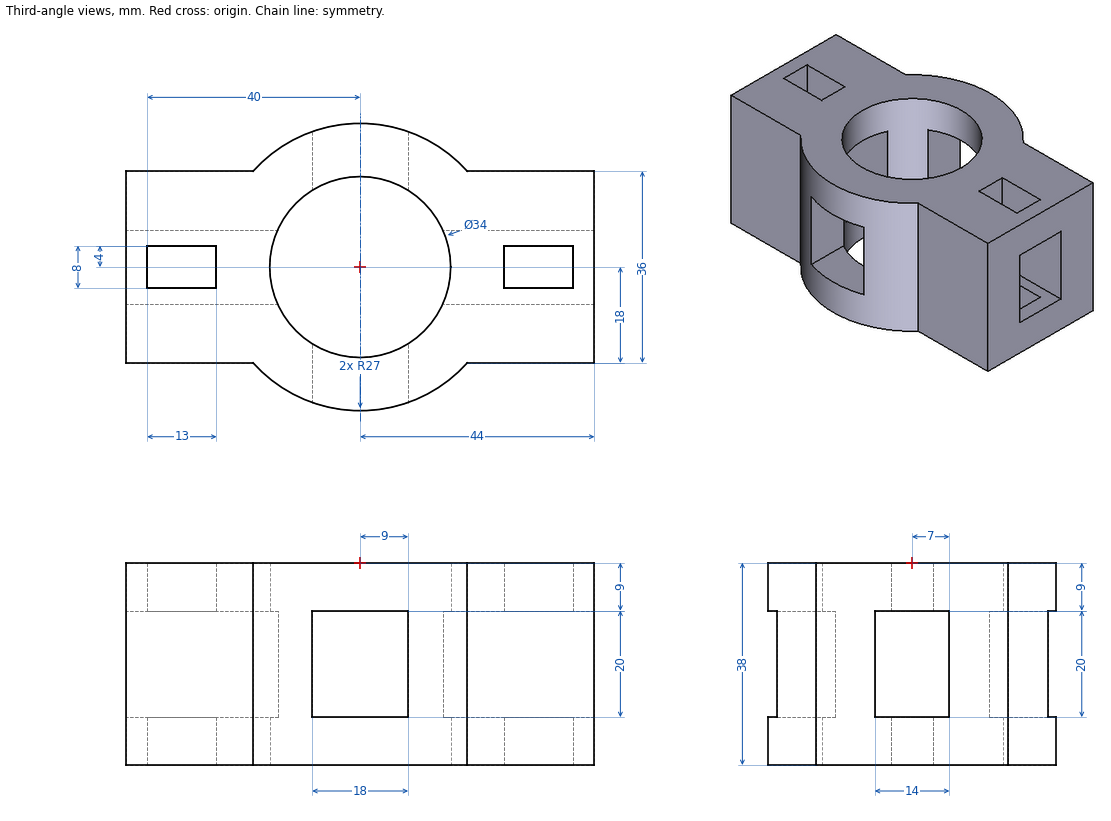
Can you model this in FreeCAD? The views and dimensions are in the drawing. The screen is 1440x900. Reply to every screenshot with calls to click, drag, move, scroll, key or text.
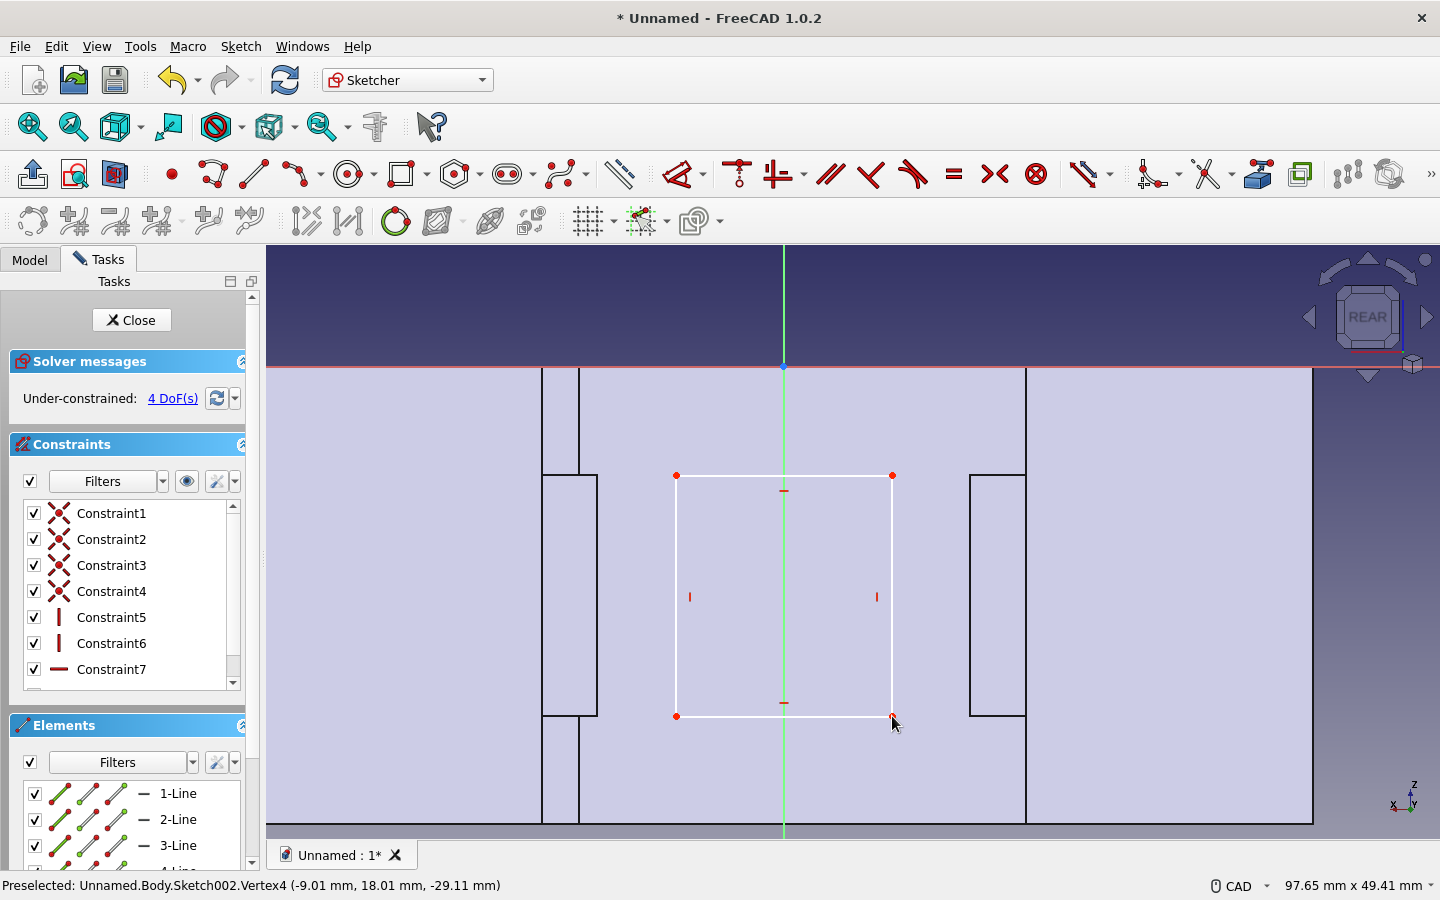
click(676, 174)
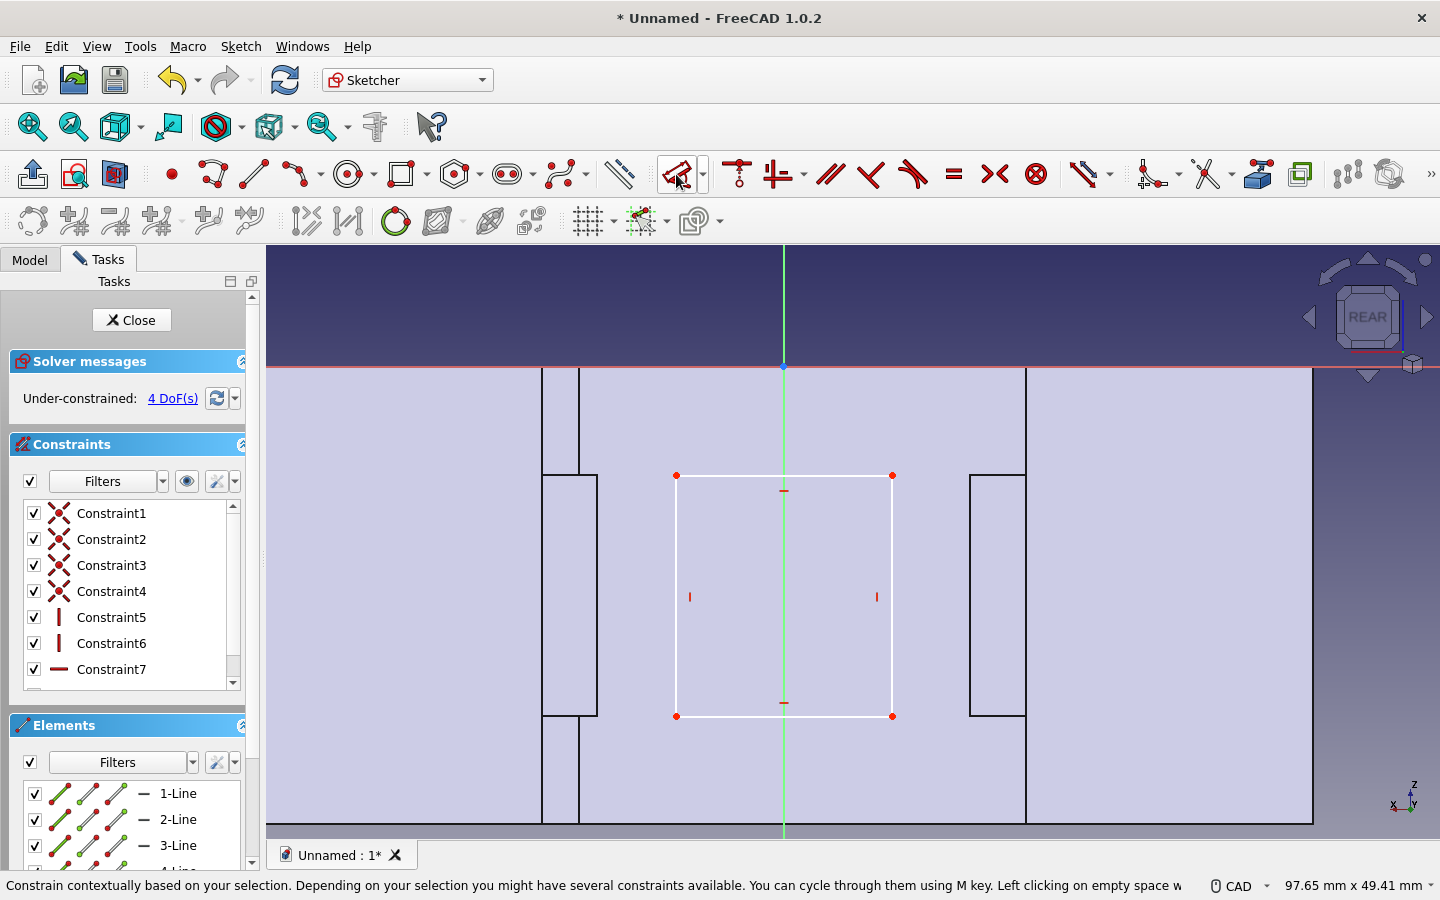
click(676, 548)
click(642, 597)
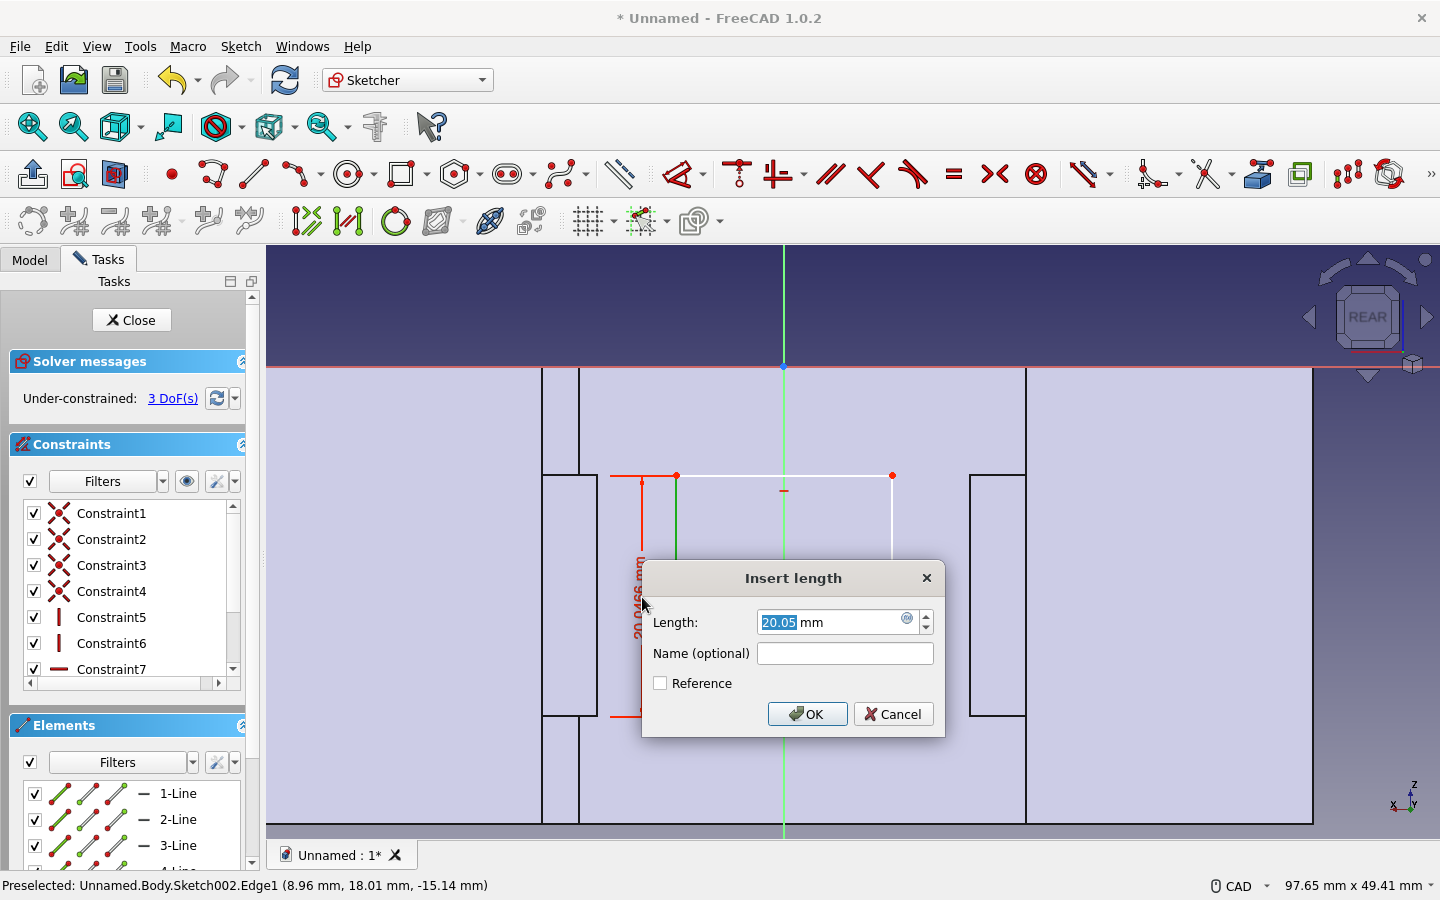
text(20)
key(Return)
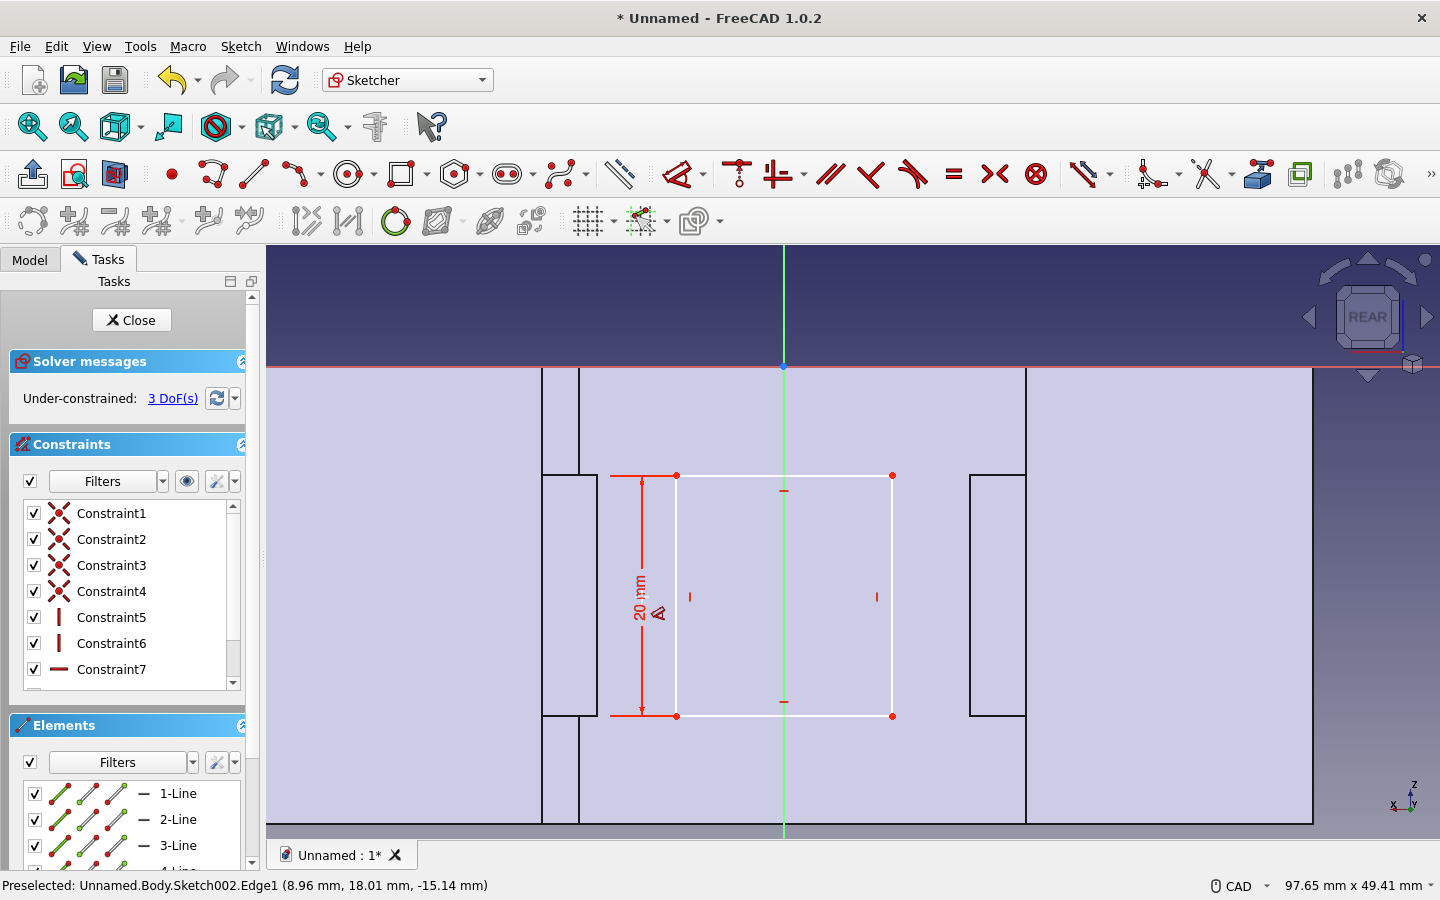
click(741, 716)
click(734, 750)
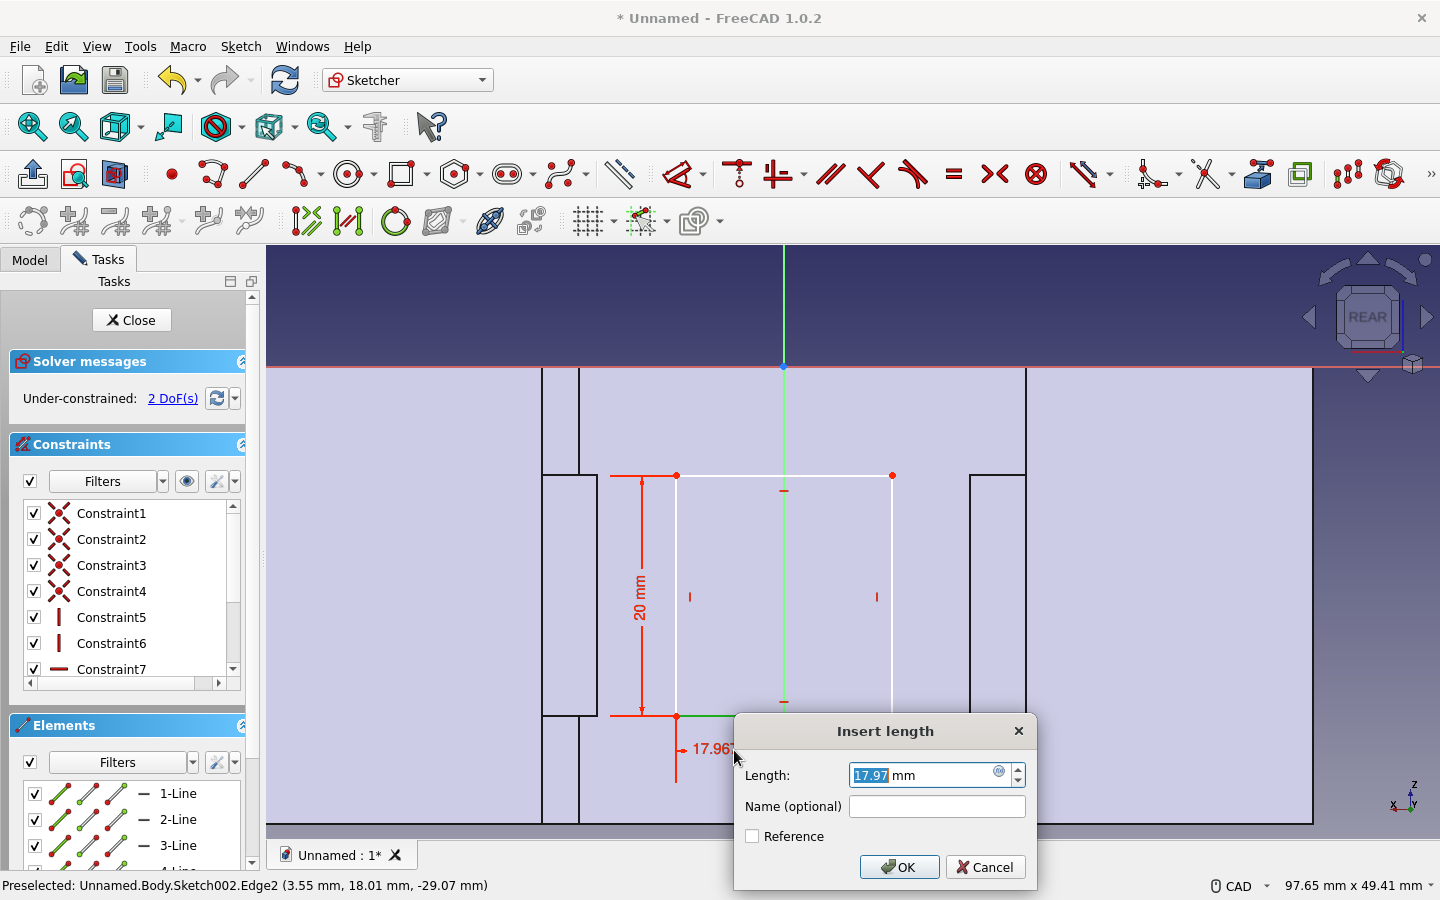
text(18)
key(Return)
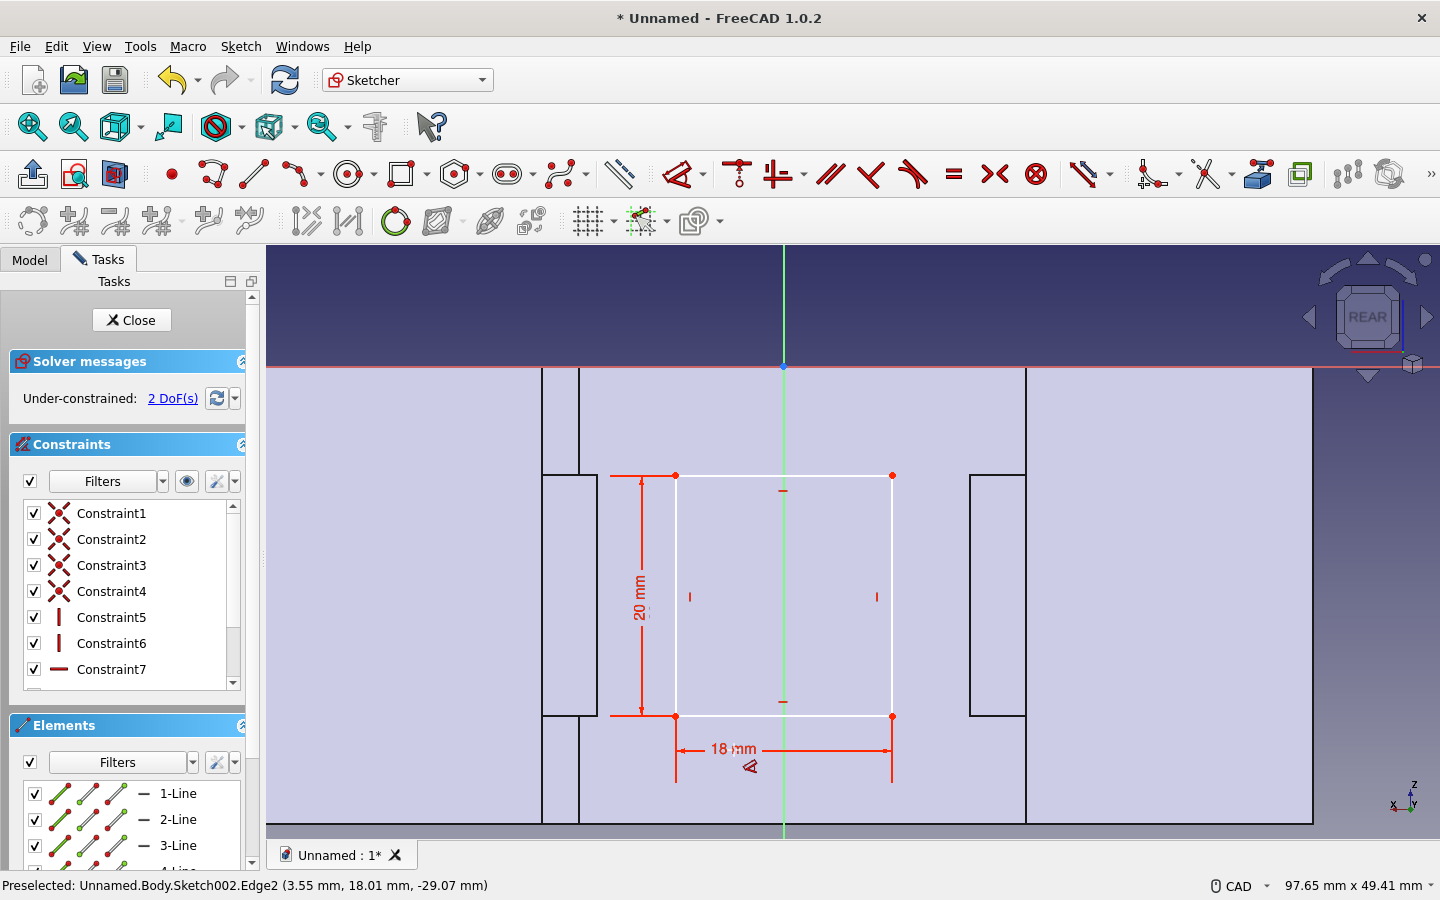
click(676, 476)
click(730, 333)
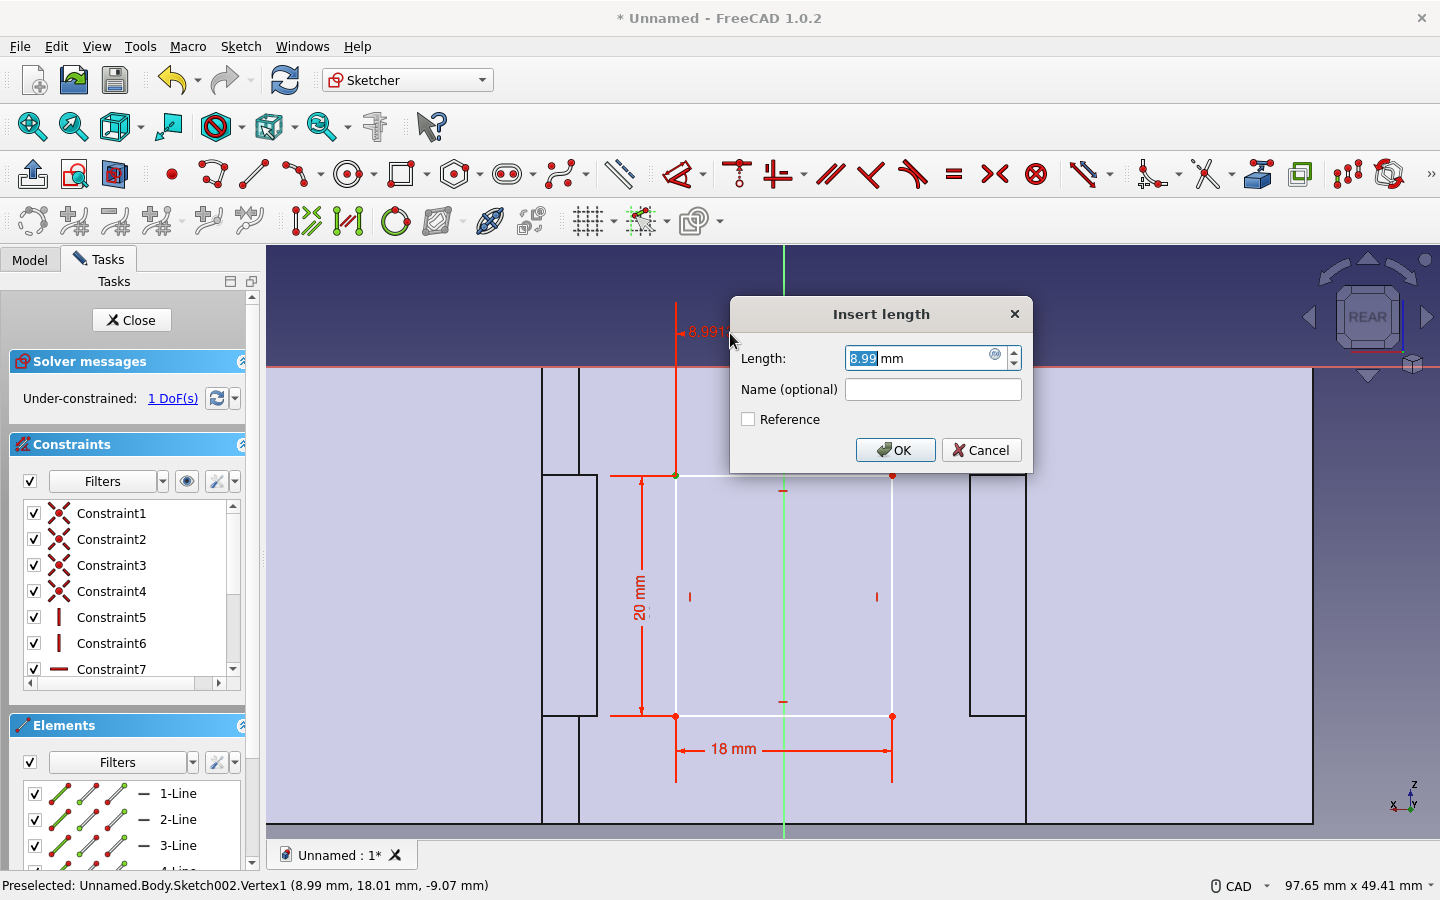
text(9)
key(Return)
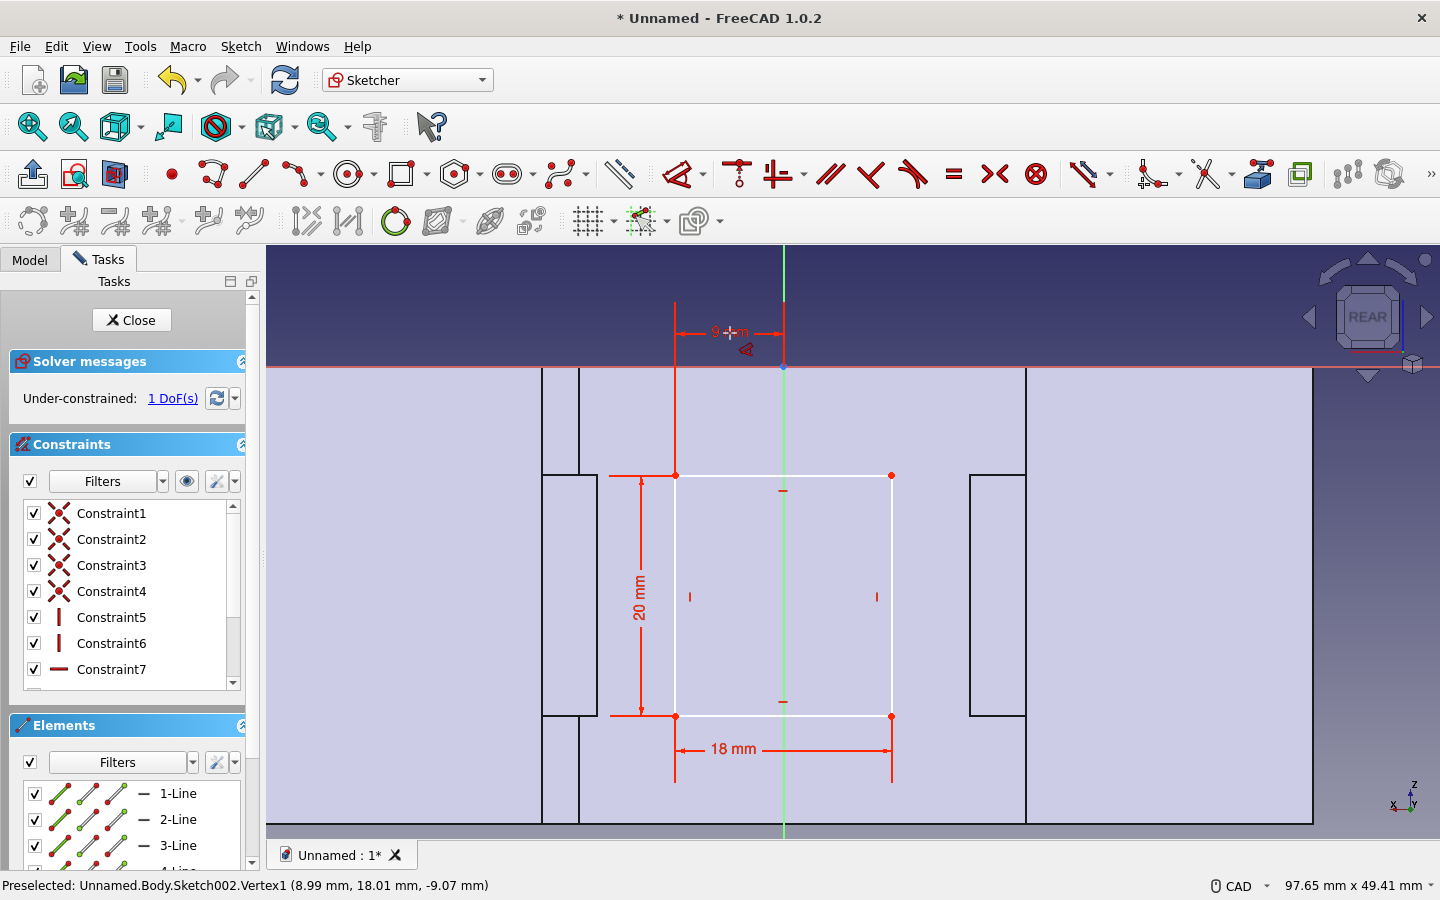
click(676, 476)
click(642, 421)